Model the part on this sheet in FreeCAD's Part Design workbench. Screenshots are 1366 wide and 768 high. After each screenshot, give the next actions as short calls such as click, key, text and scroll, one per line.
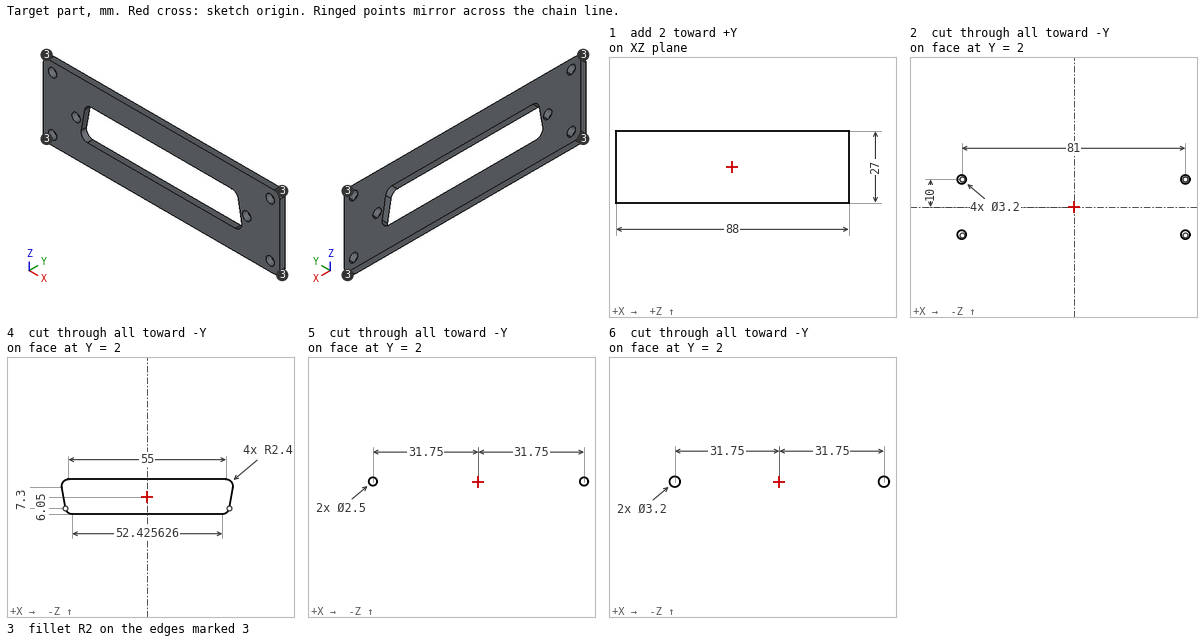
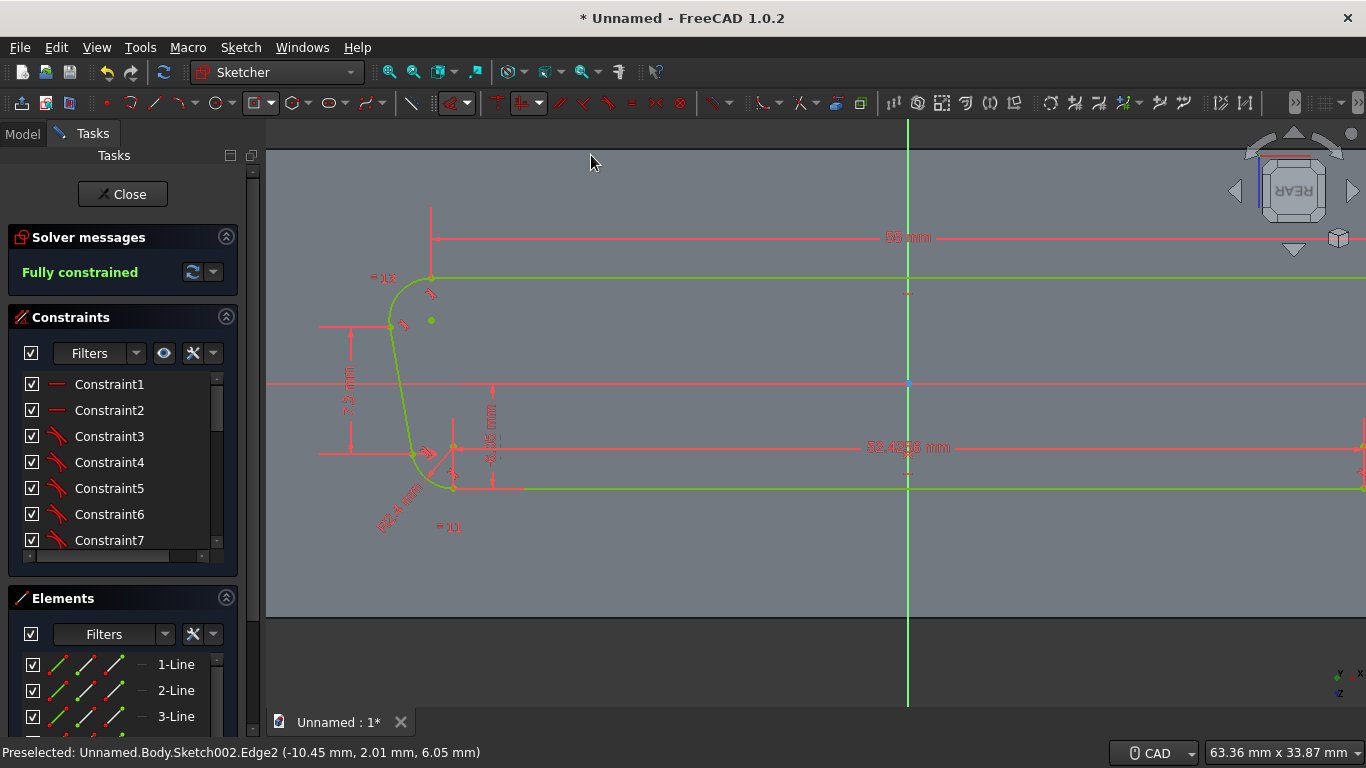
click(123, 194)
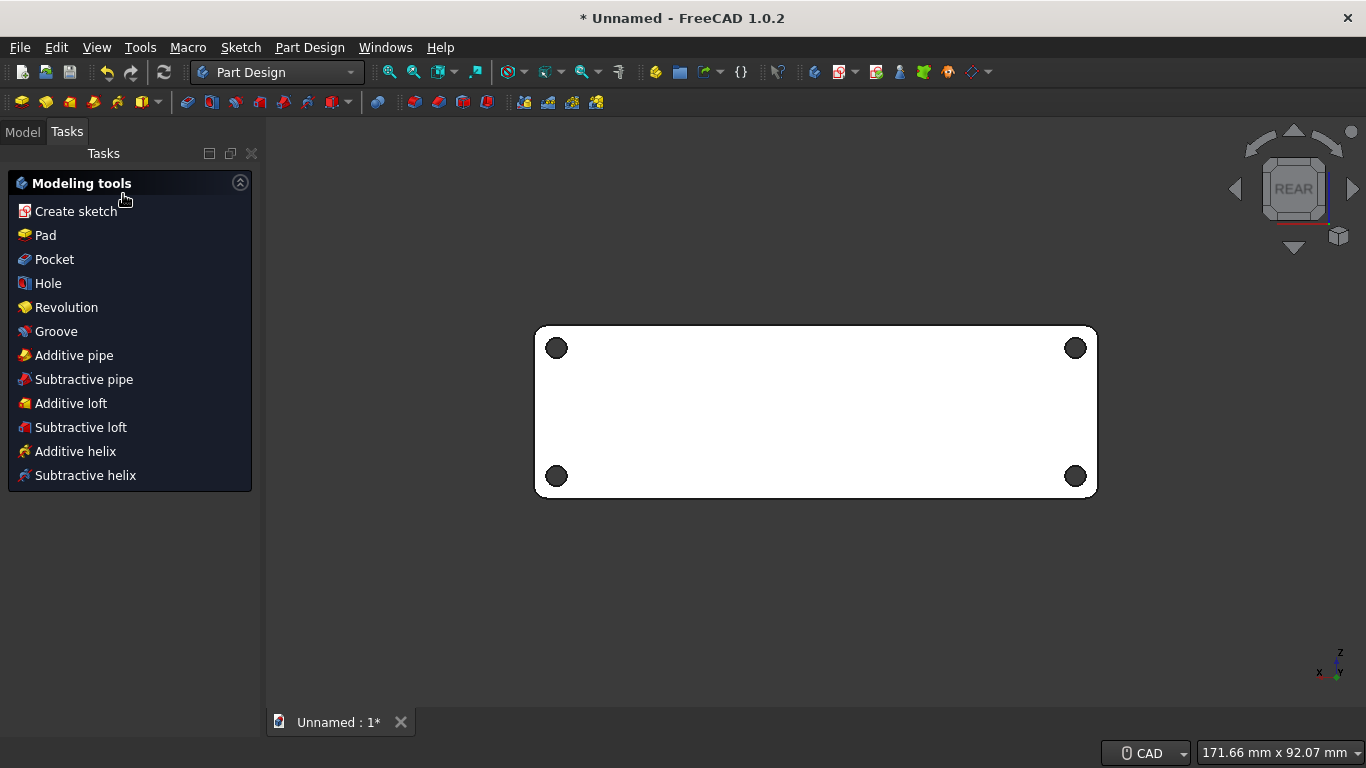
click(188, 102)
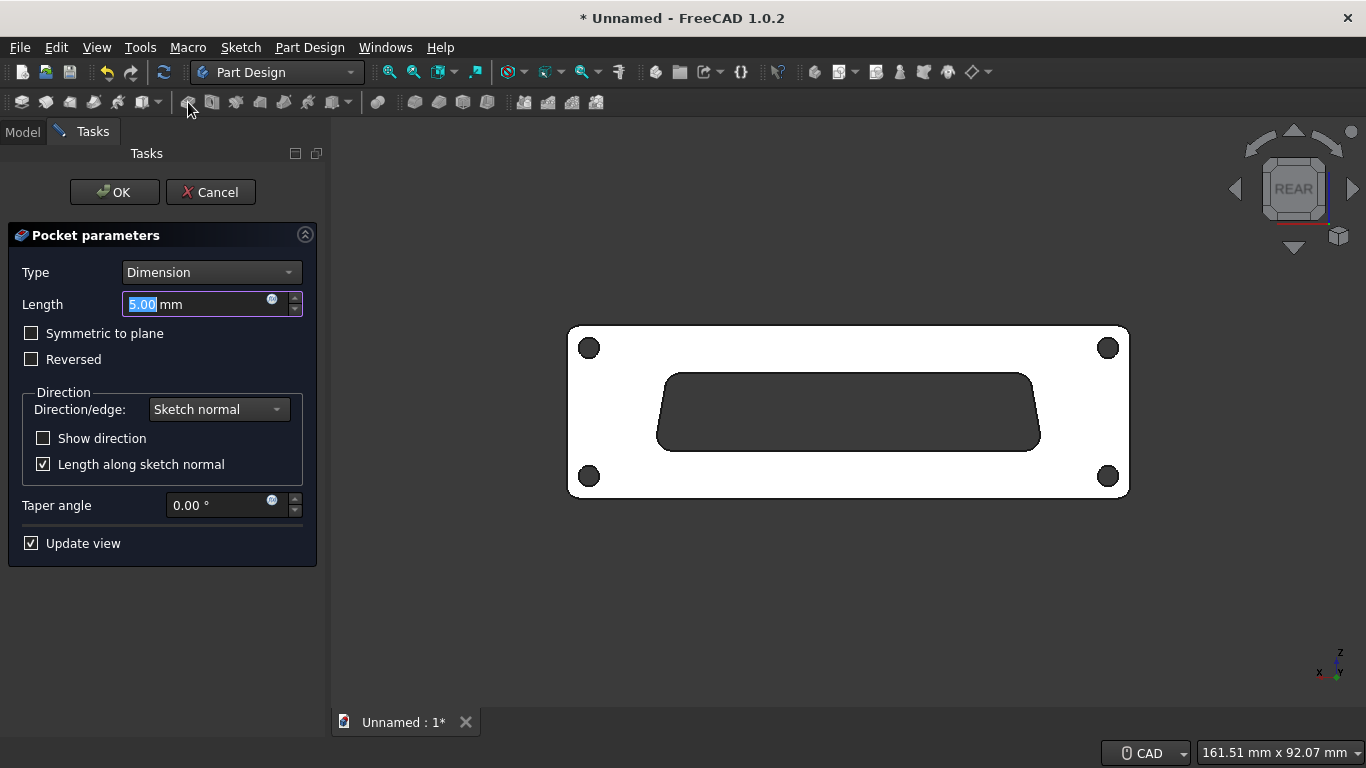
click(212, 272)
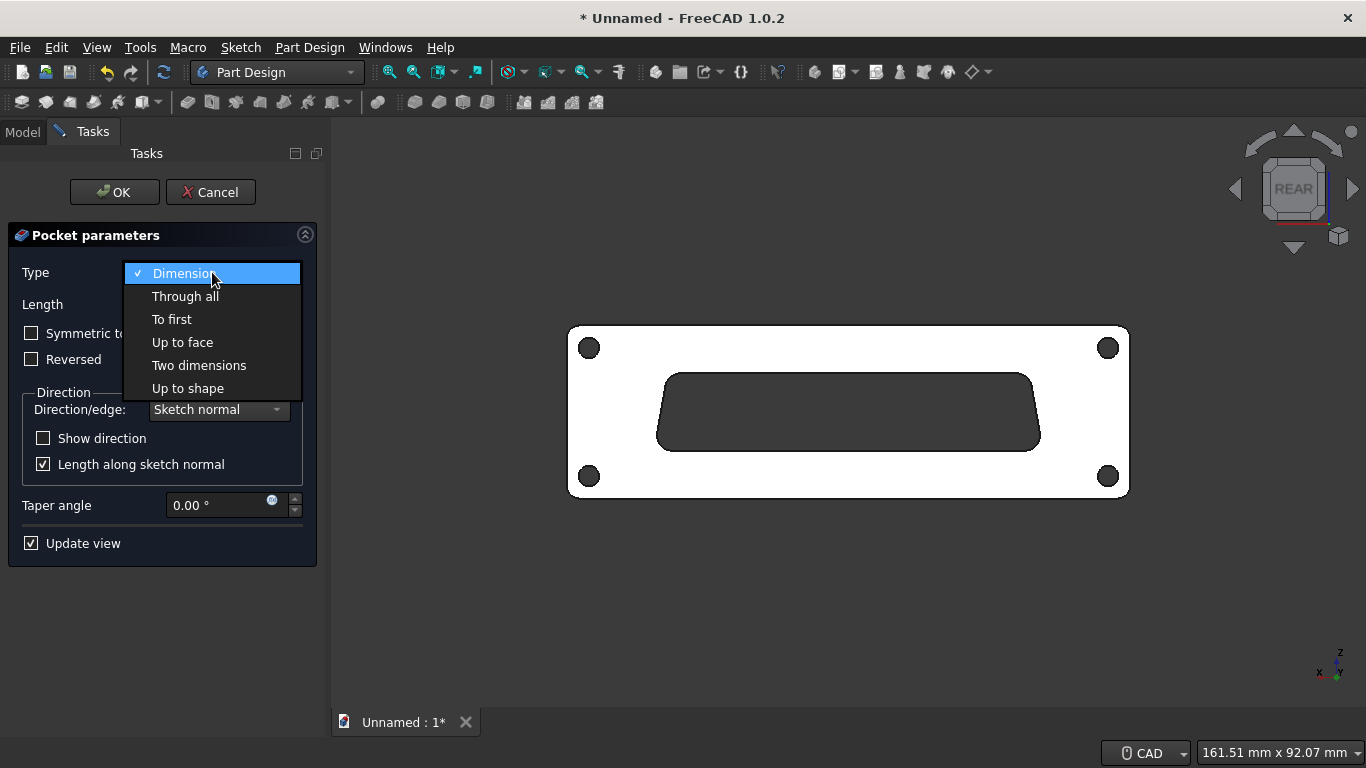
click(212, 296)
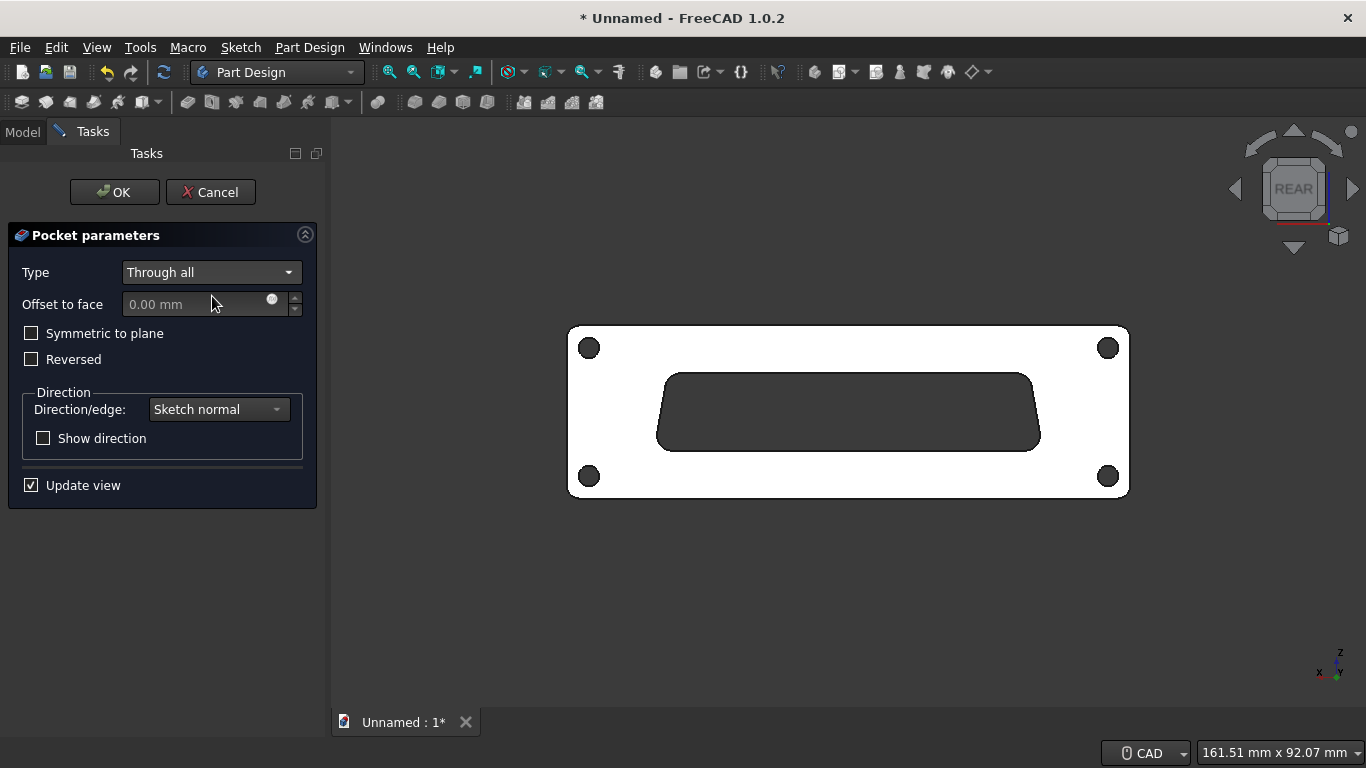
click(115, 192)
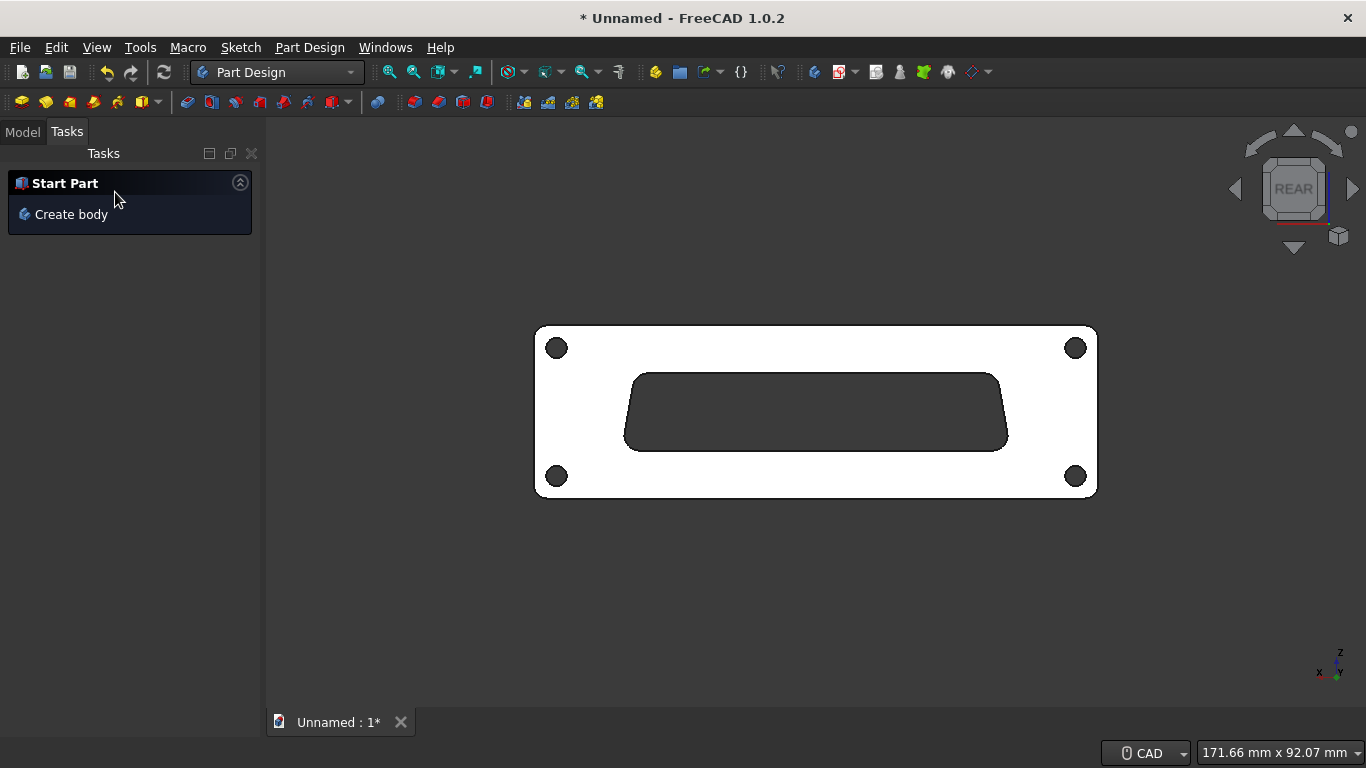
click(1058, 411)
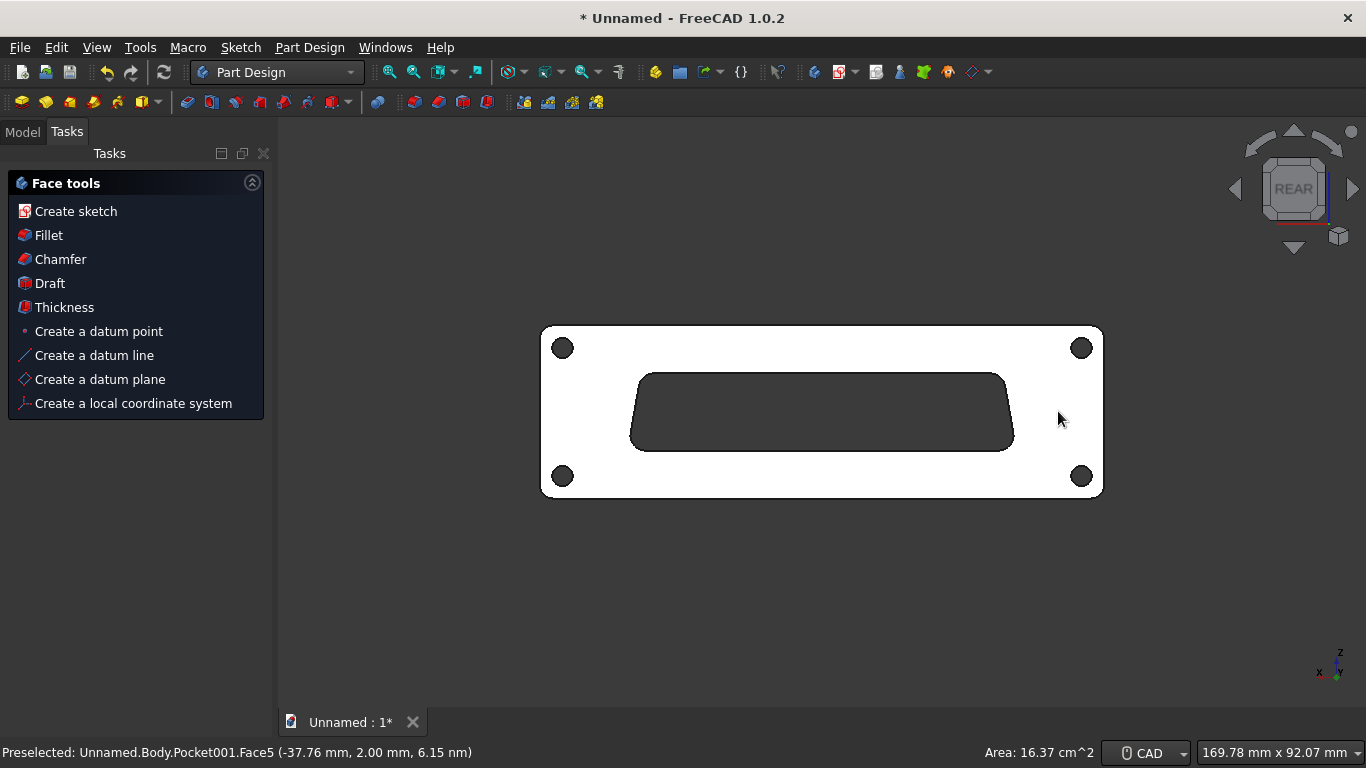
click(840, 72)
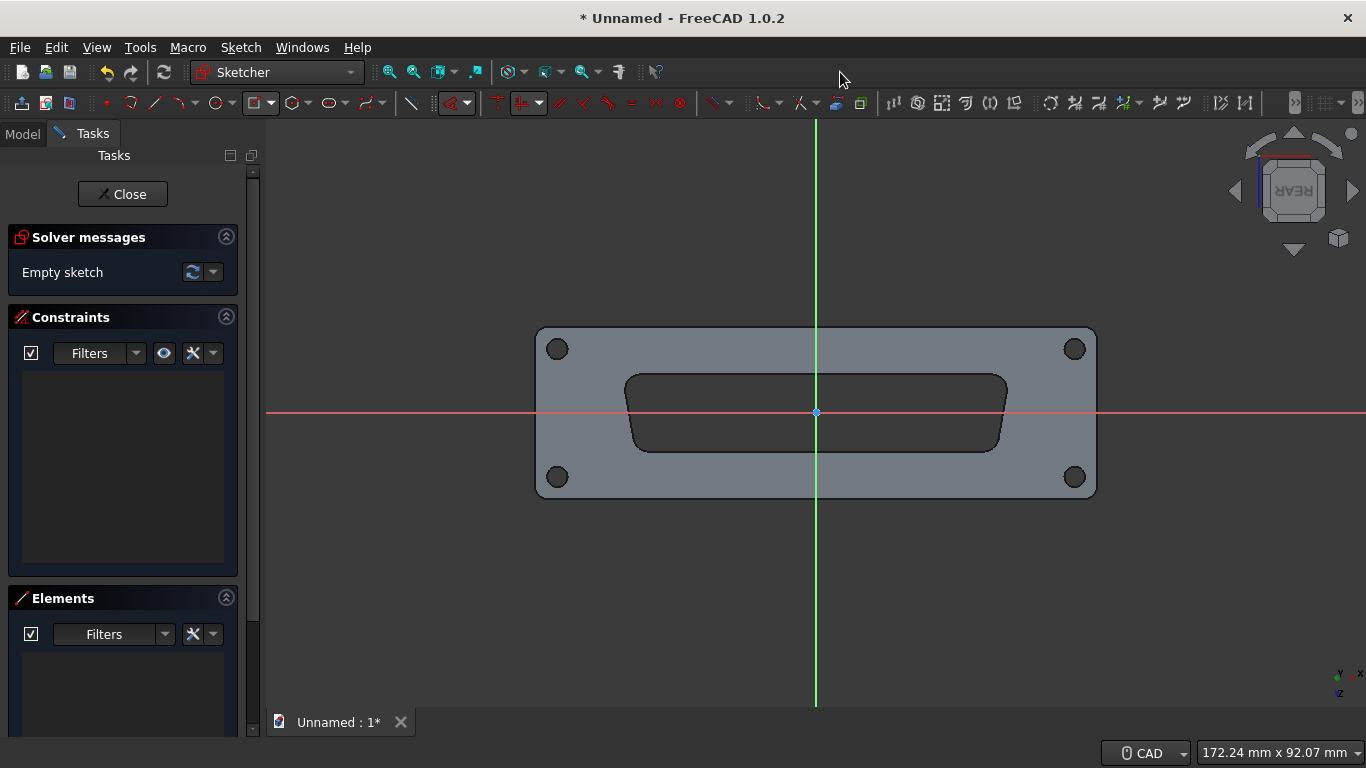
scroll(955, 413, up, 2)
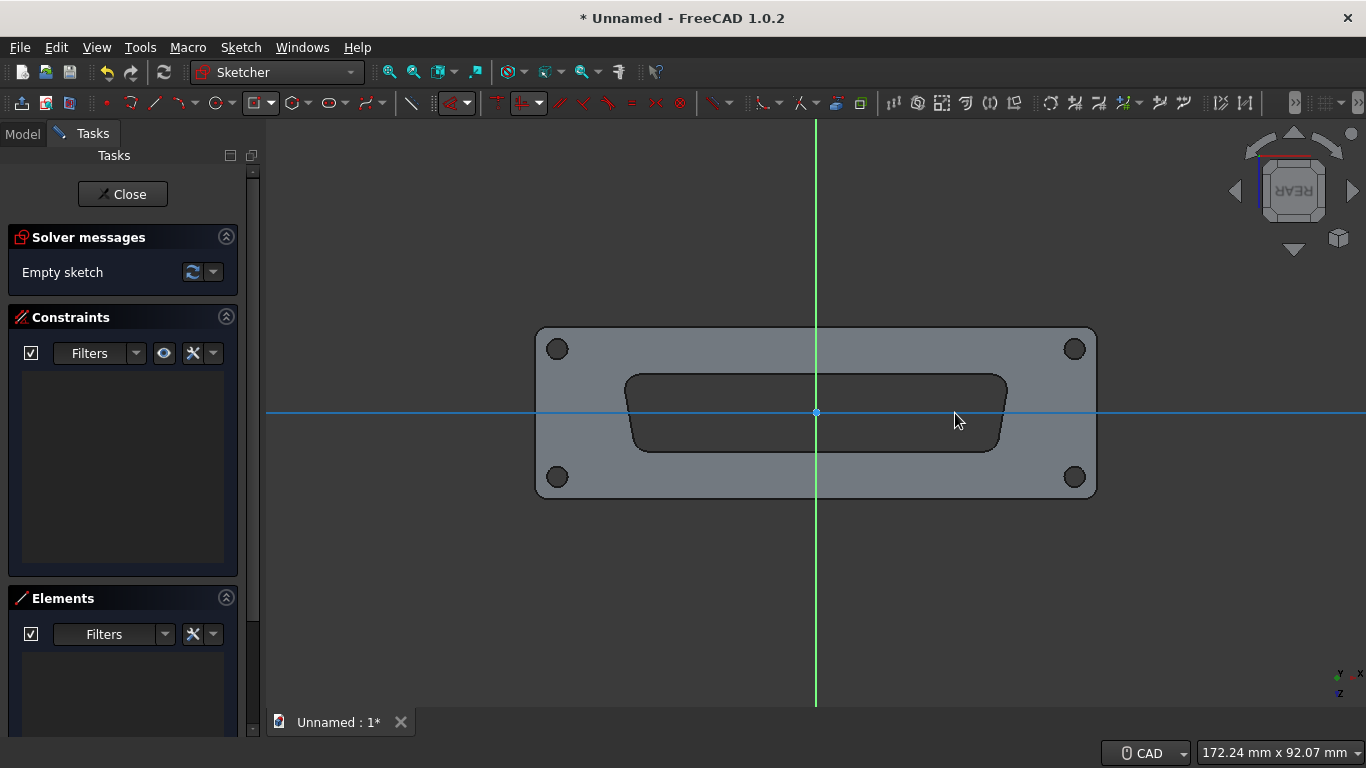
click(216, 104)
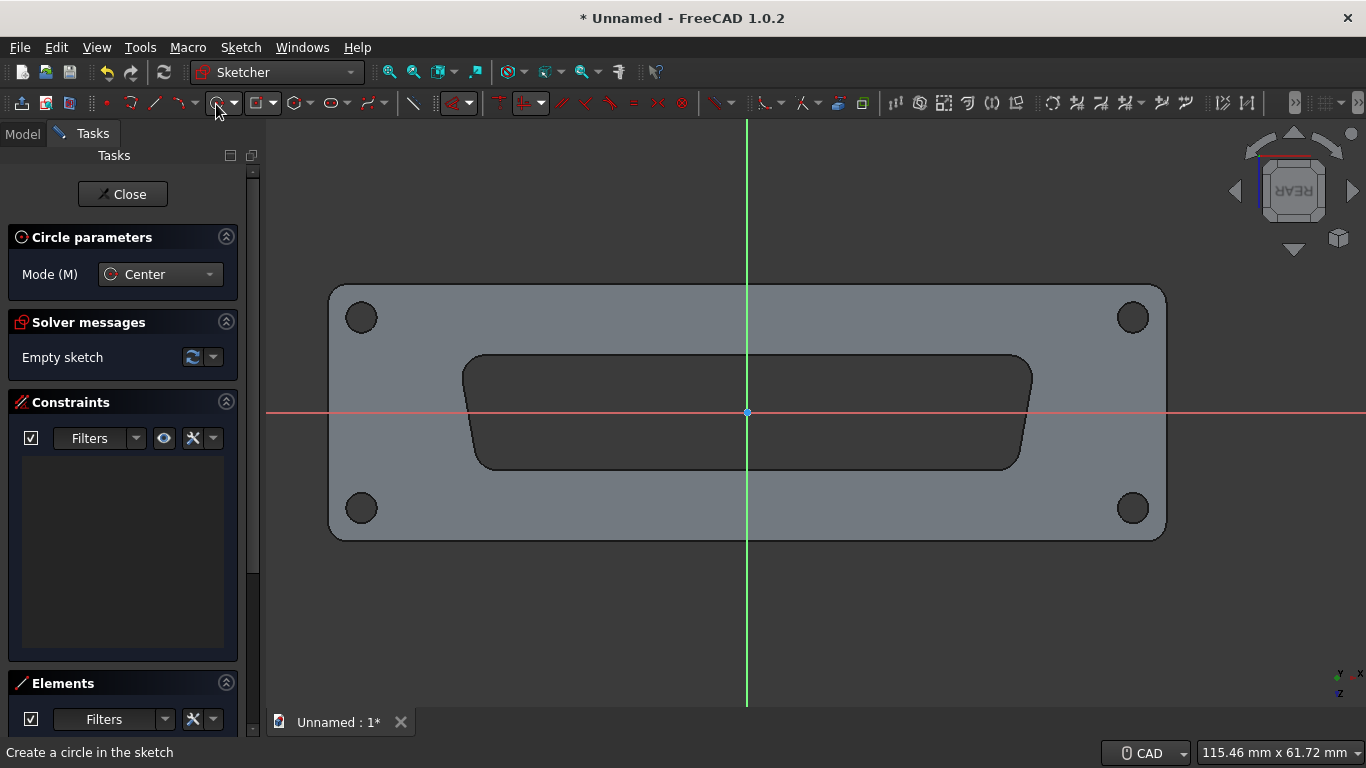
scroll(445, 413, up, 4)